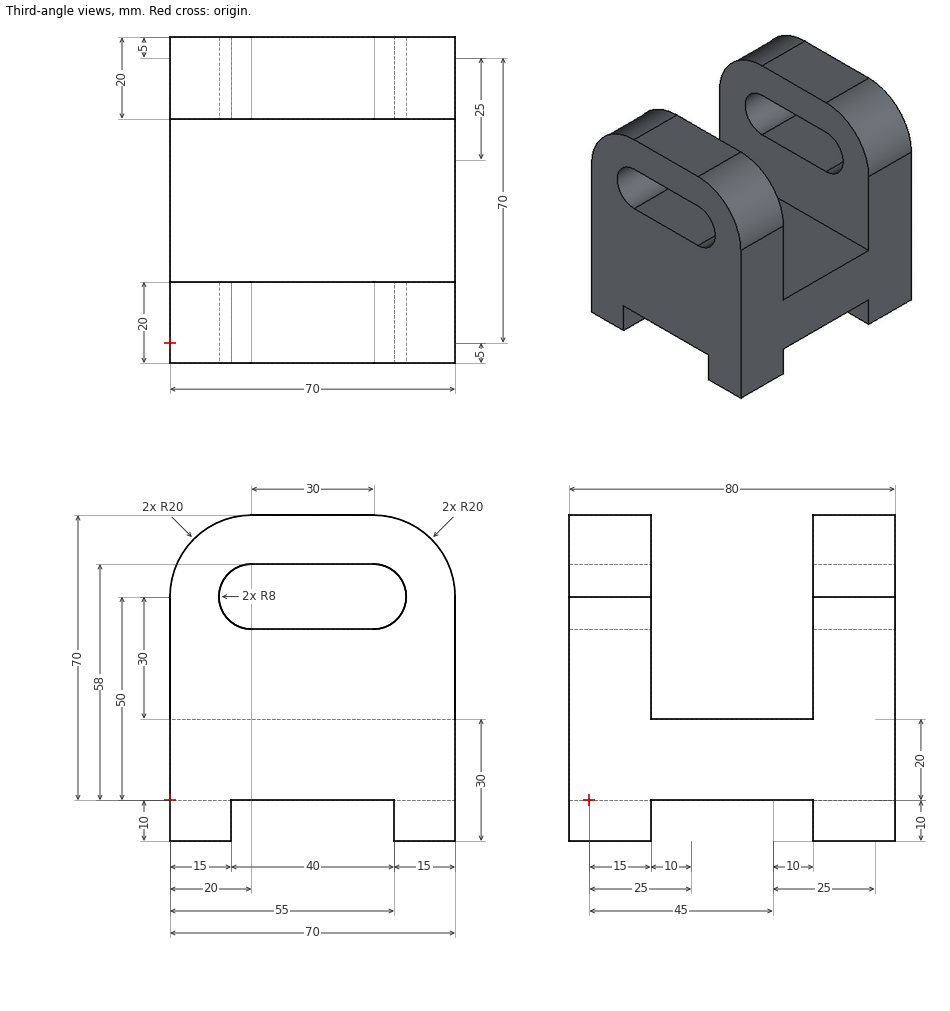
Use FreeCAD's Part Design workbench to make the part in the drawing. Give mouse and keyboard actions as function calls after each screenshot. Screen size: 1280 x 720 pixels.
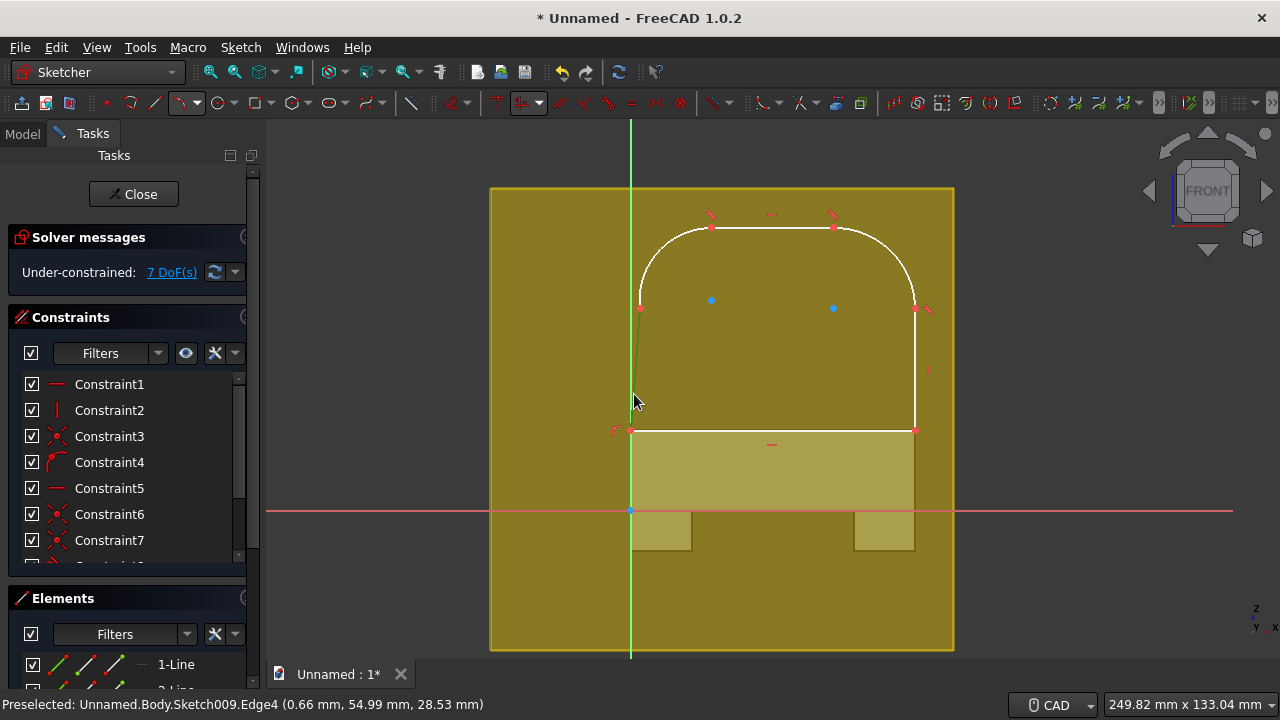
click(677, 237)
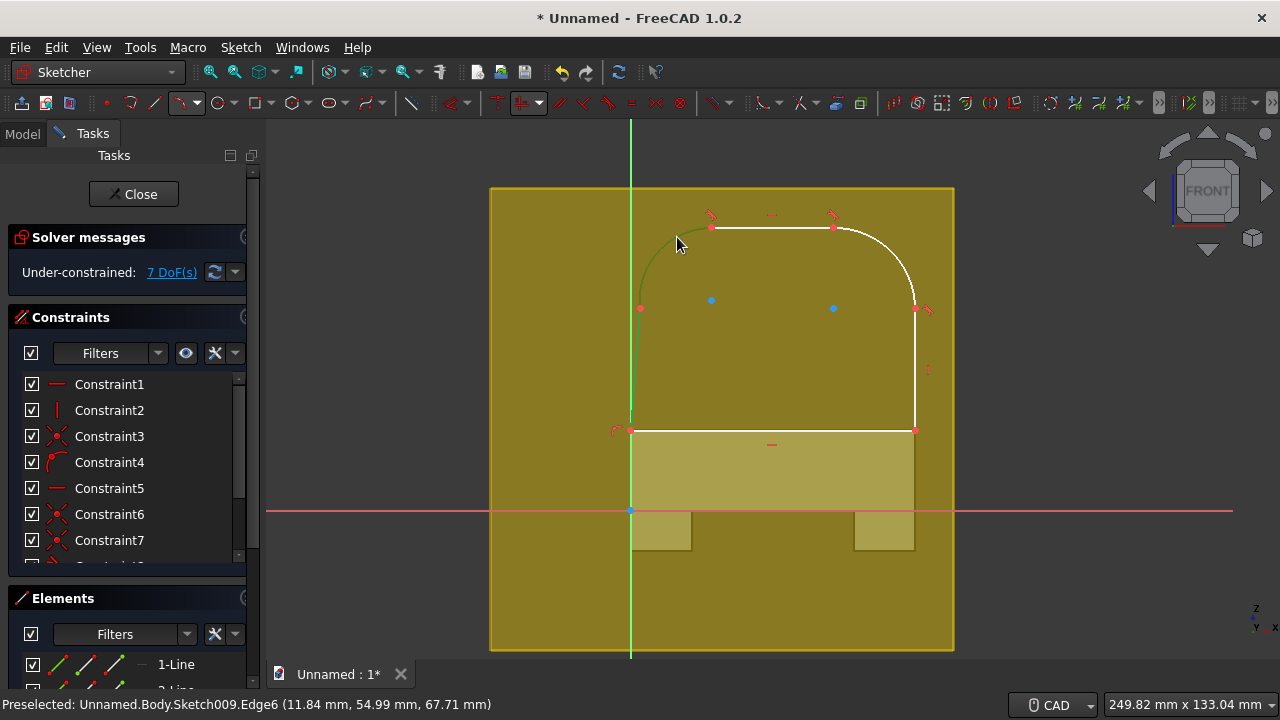
key(t)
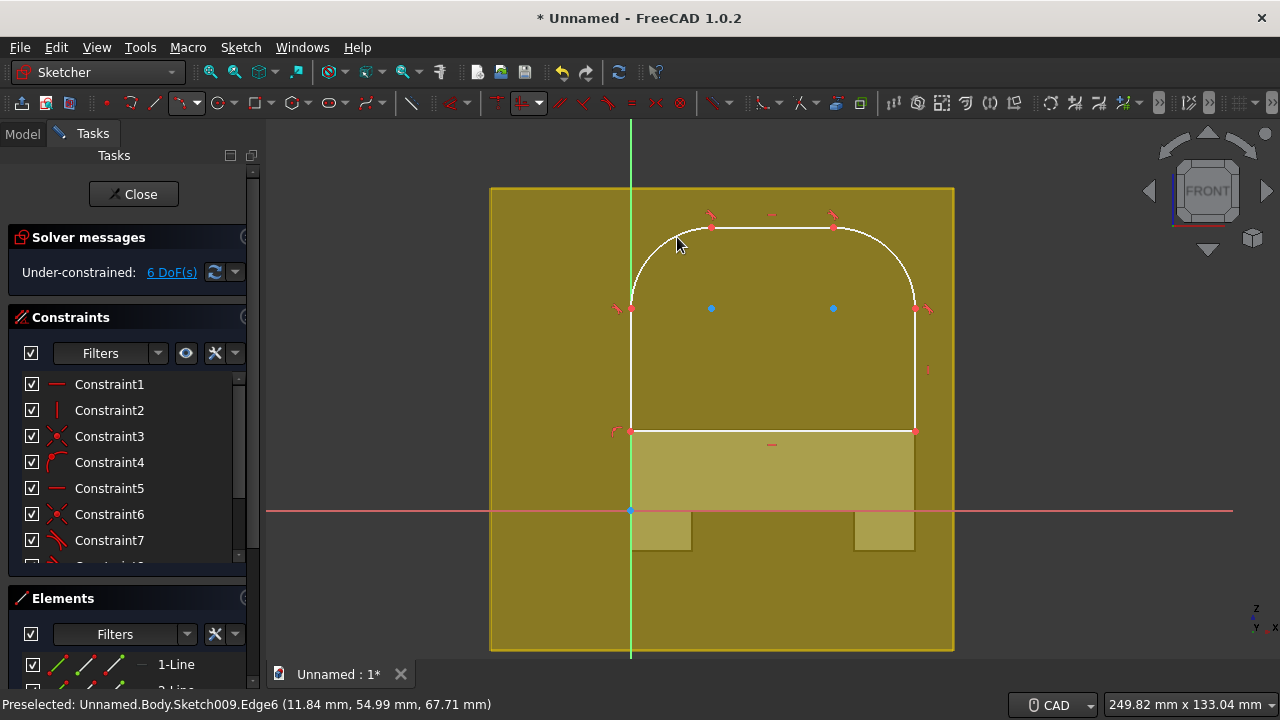
click(631, 394)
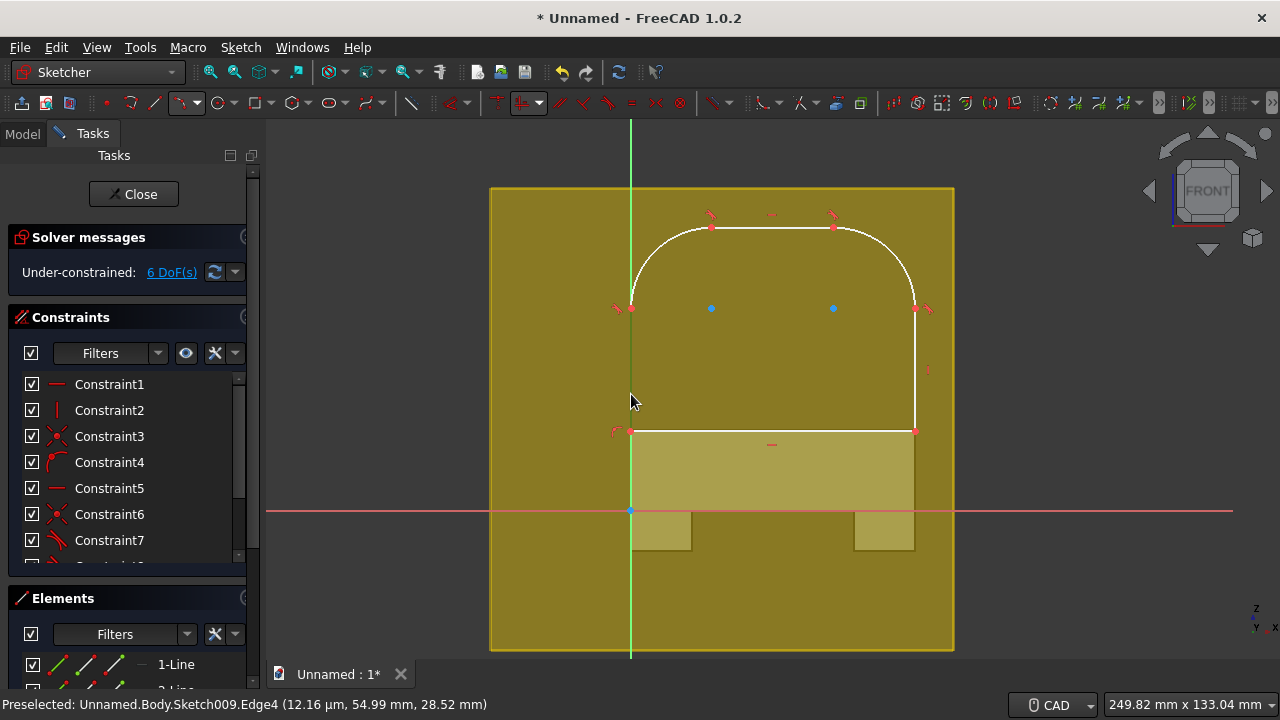
key(v)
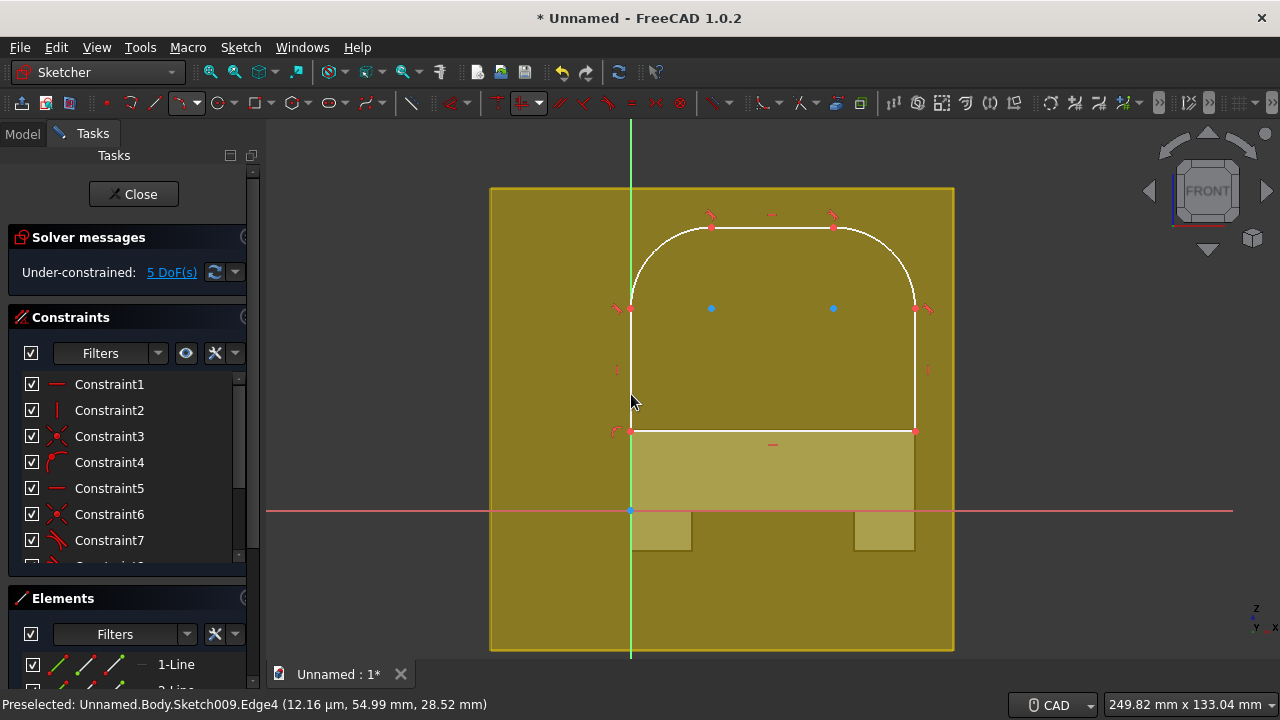
click(906, 272)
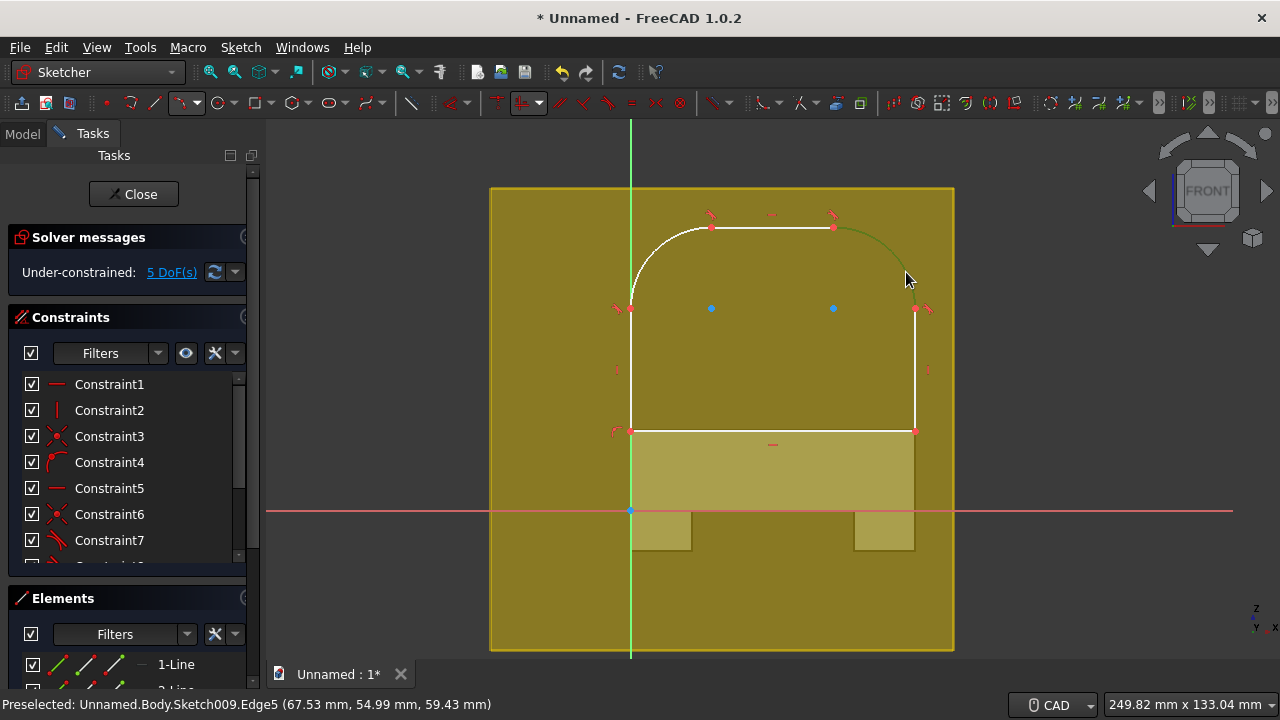
click(675, 236)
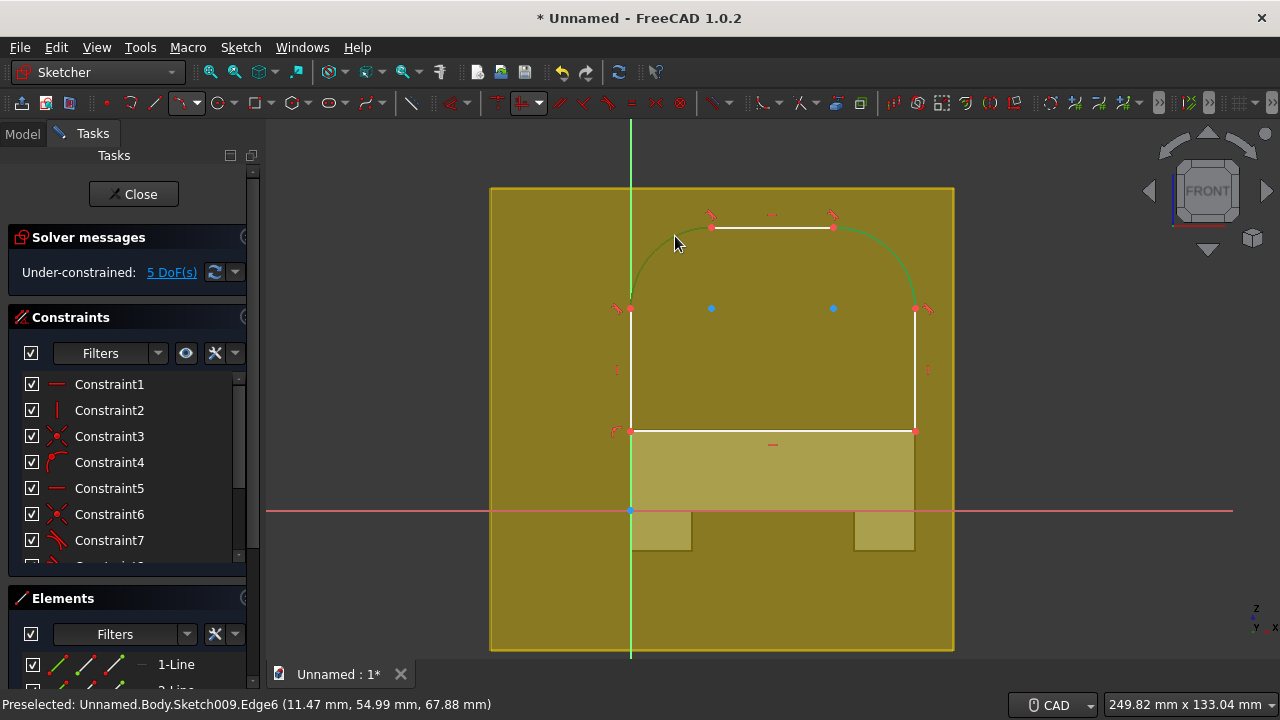
key(e)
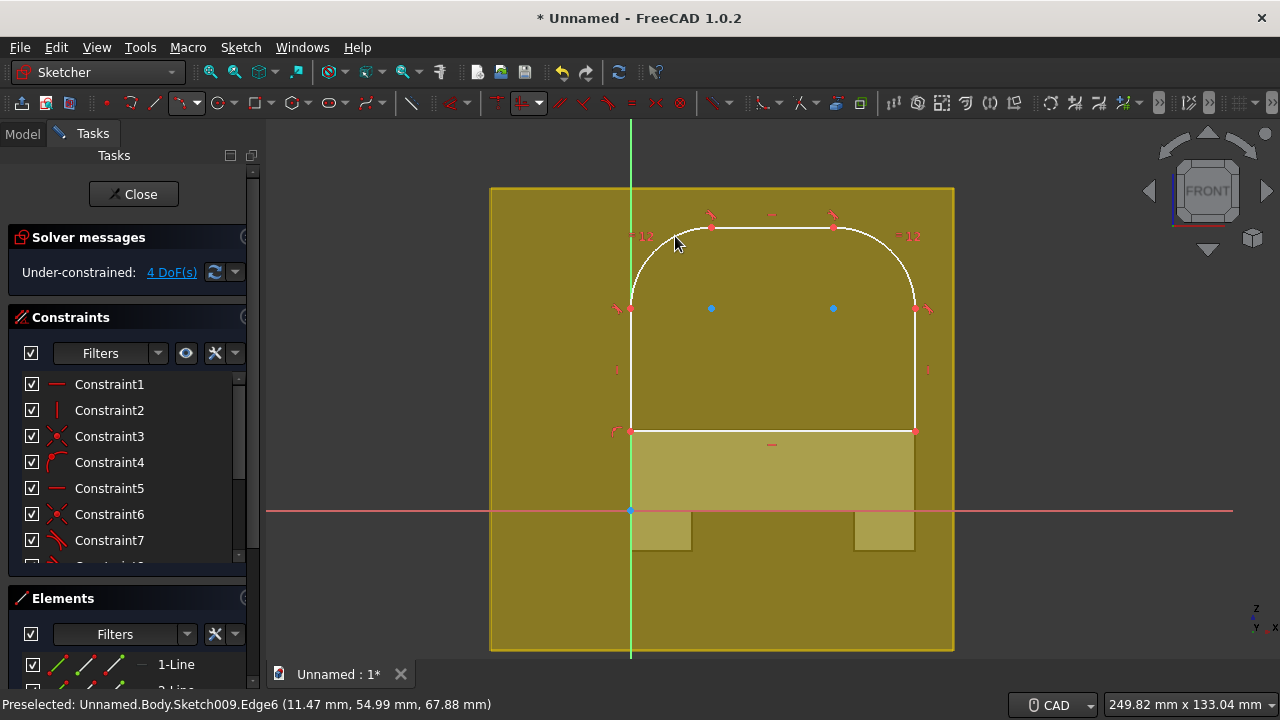
click(450, 104)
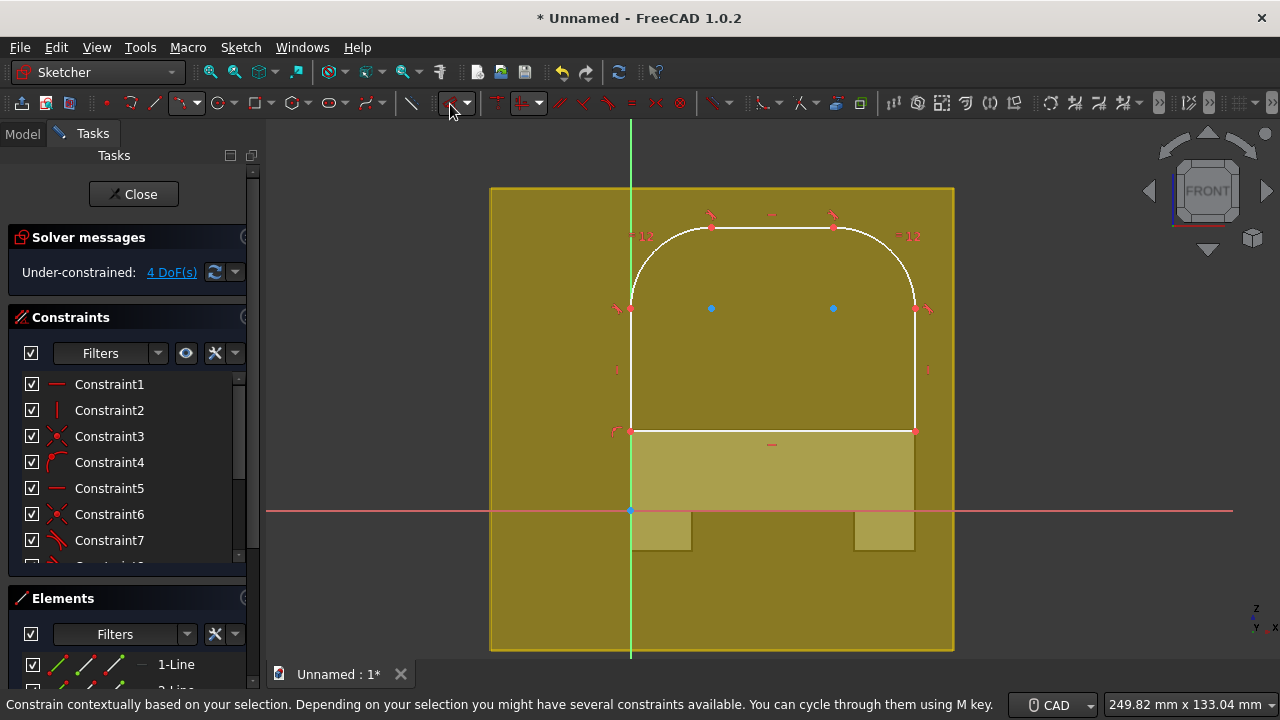
click(906, 272)
click(935, 258)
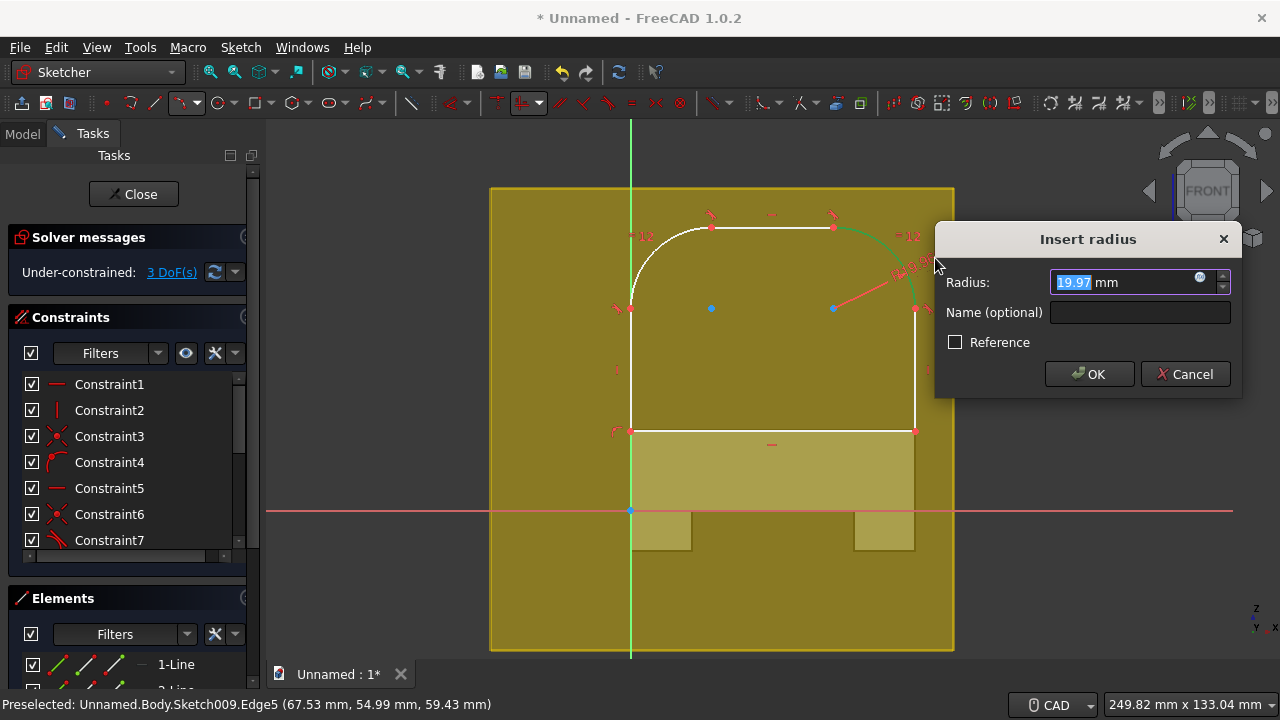
text(20)
key(Return)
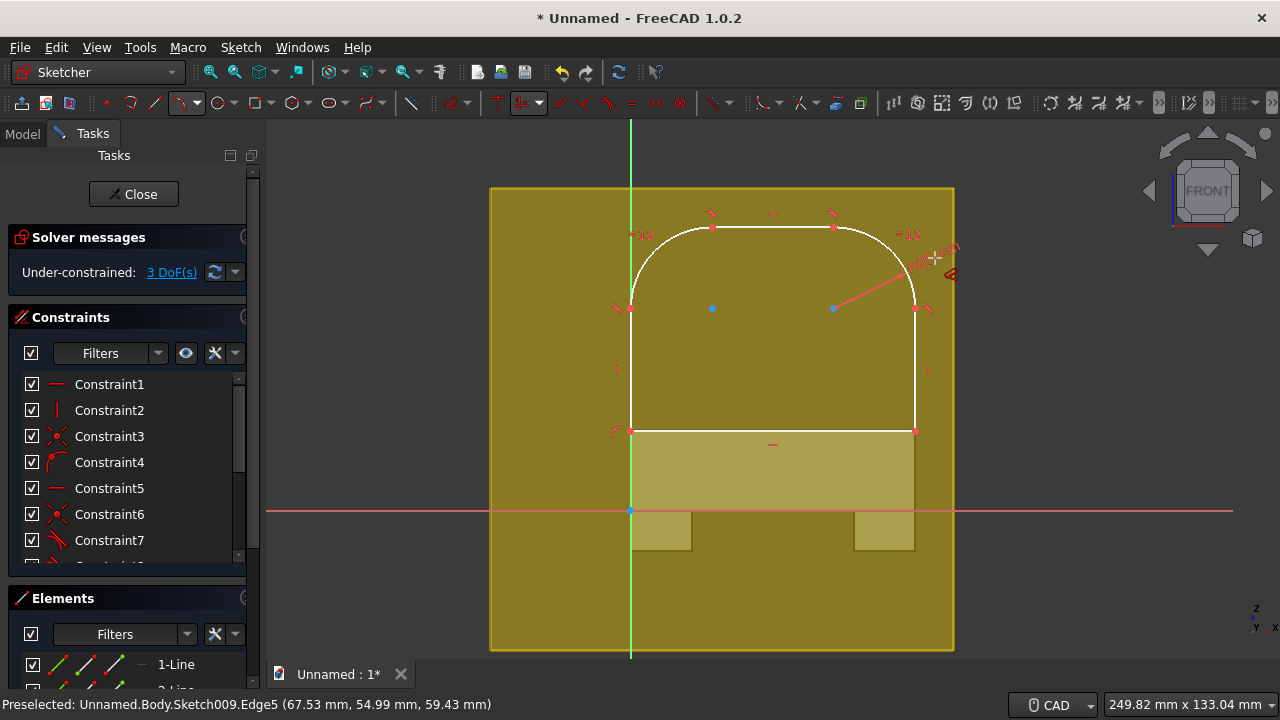
click(749, 227)
click(773, 193)